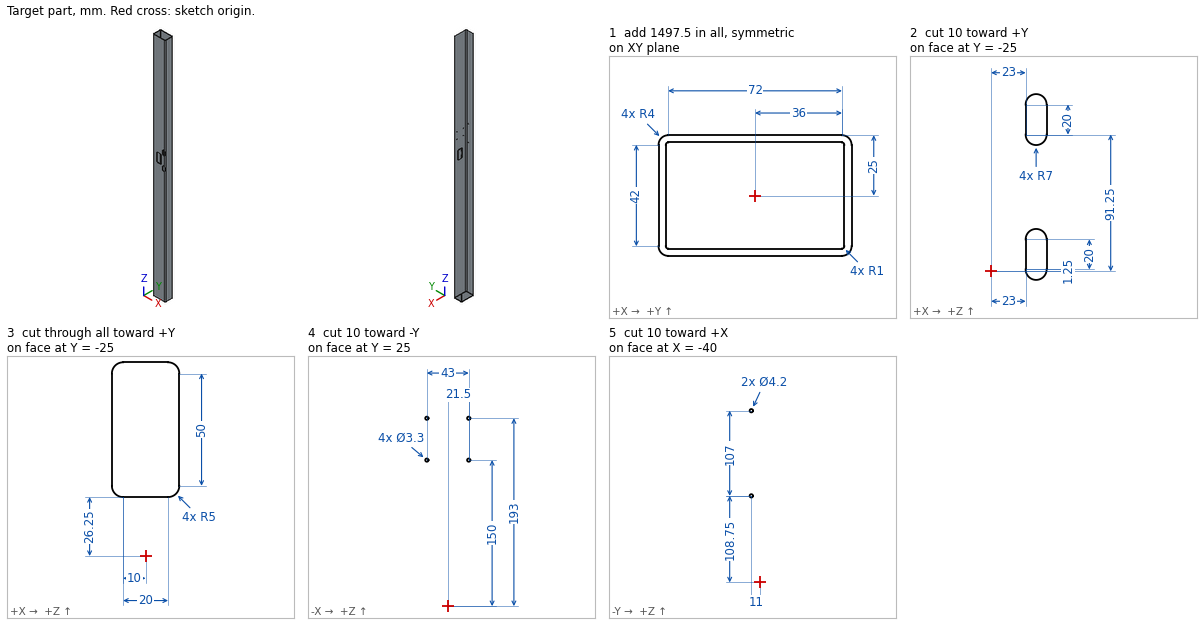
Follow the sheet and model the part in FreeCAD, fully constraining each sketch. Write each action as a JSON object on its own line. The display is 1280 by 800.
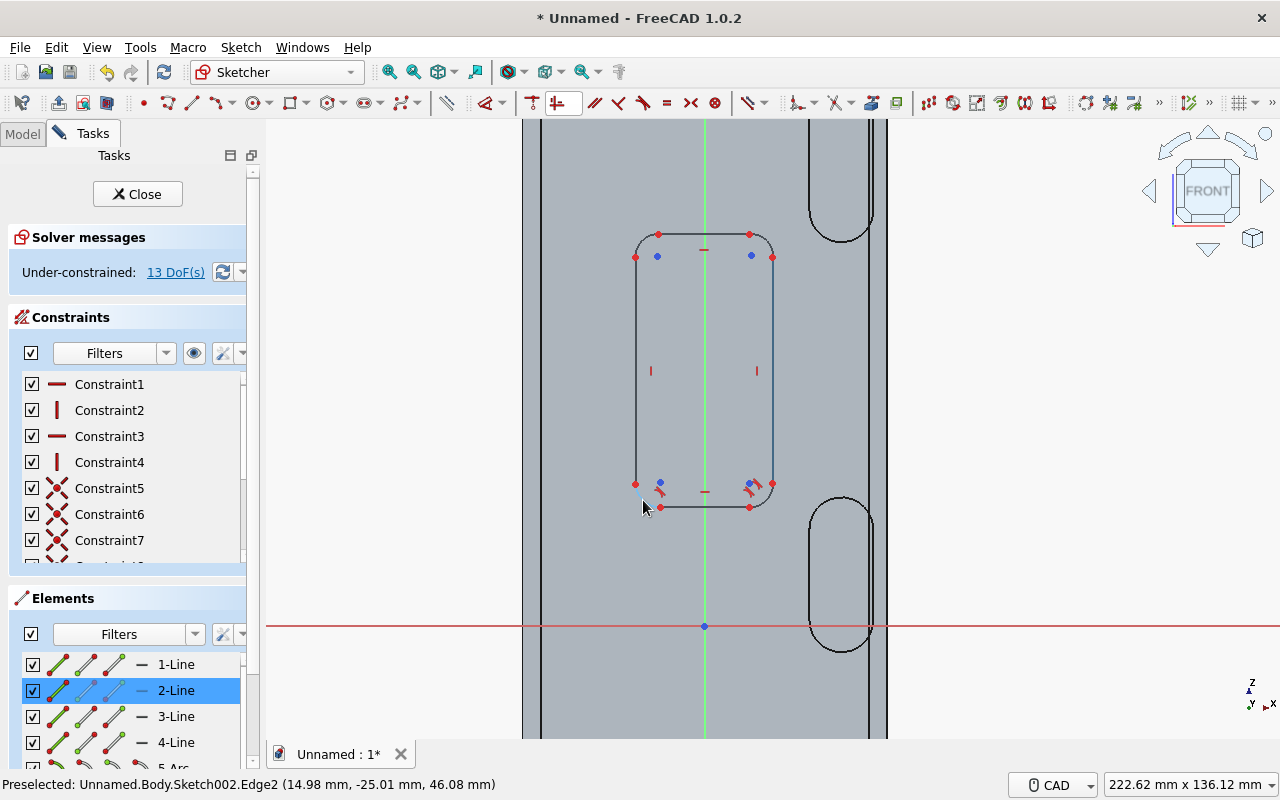
{"action": "scroll", "coordinate": [771, 247], "scroll_direction": "up", "scroll_amount": 2}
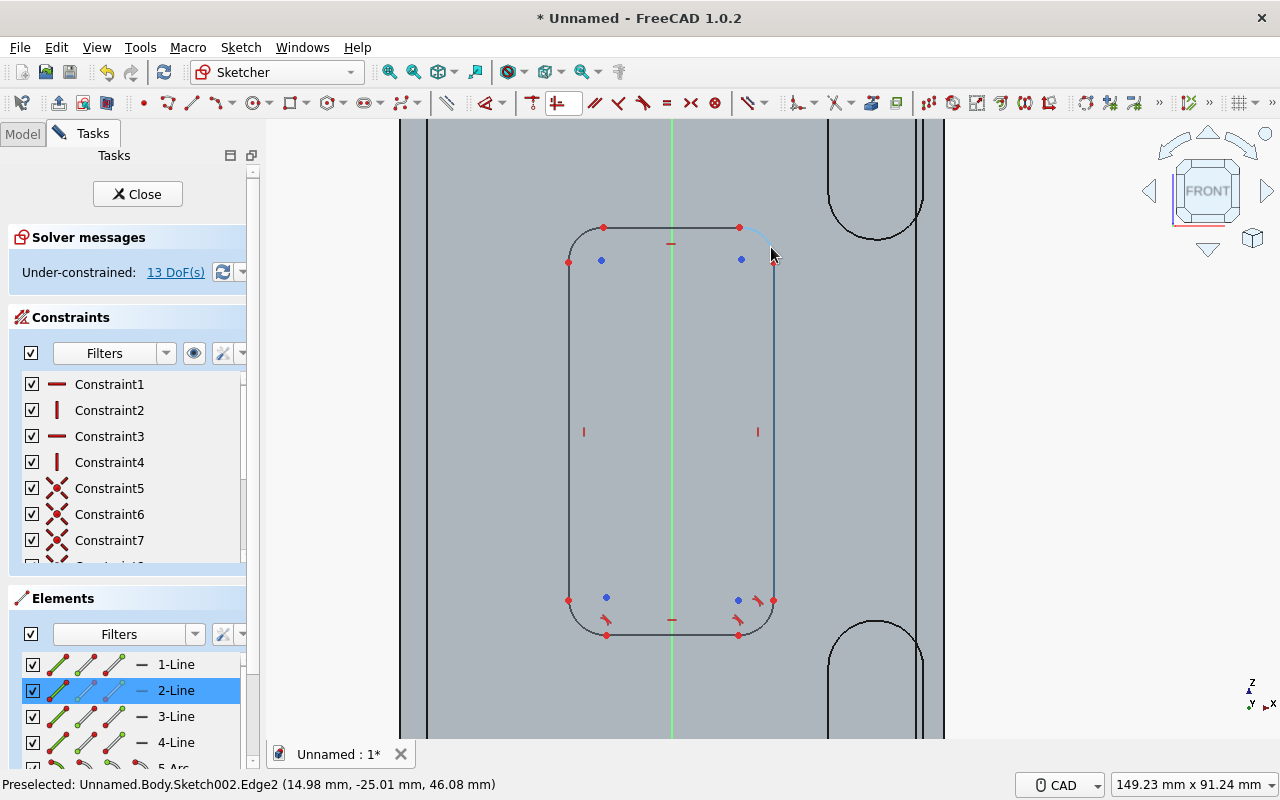
{"action": "left_click", "coordinate": [771, 246]}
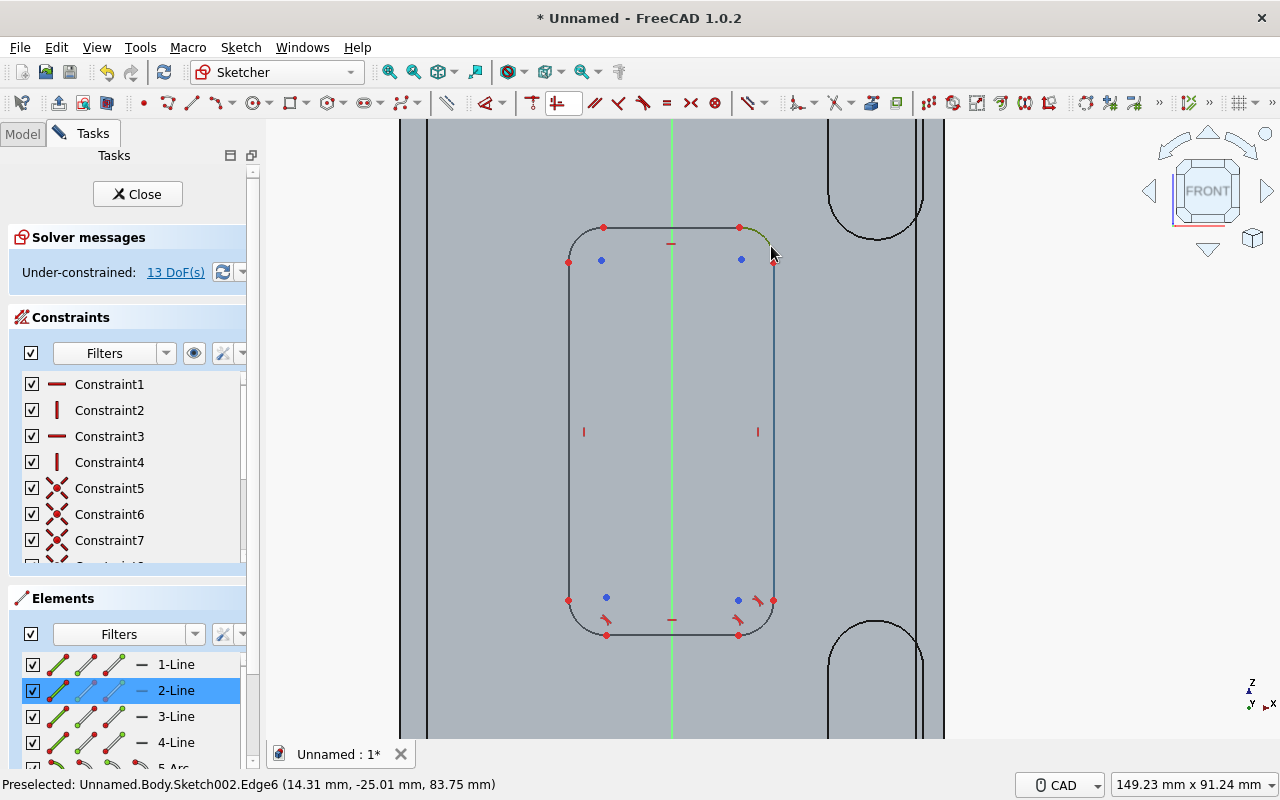
{"action": "key", "text": "t"}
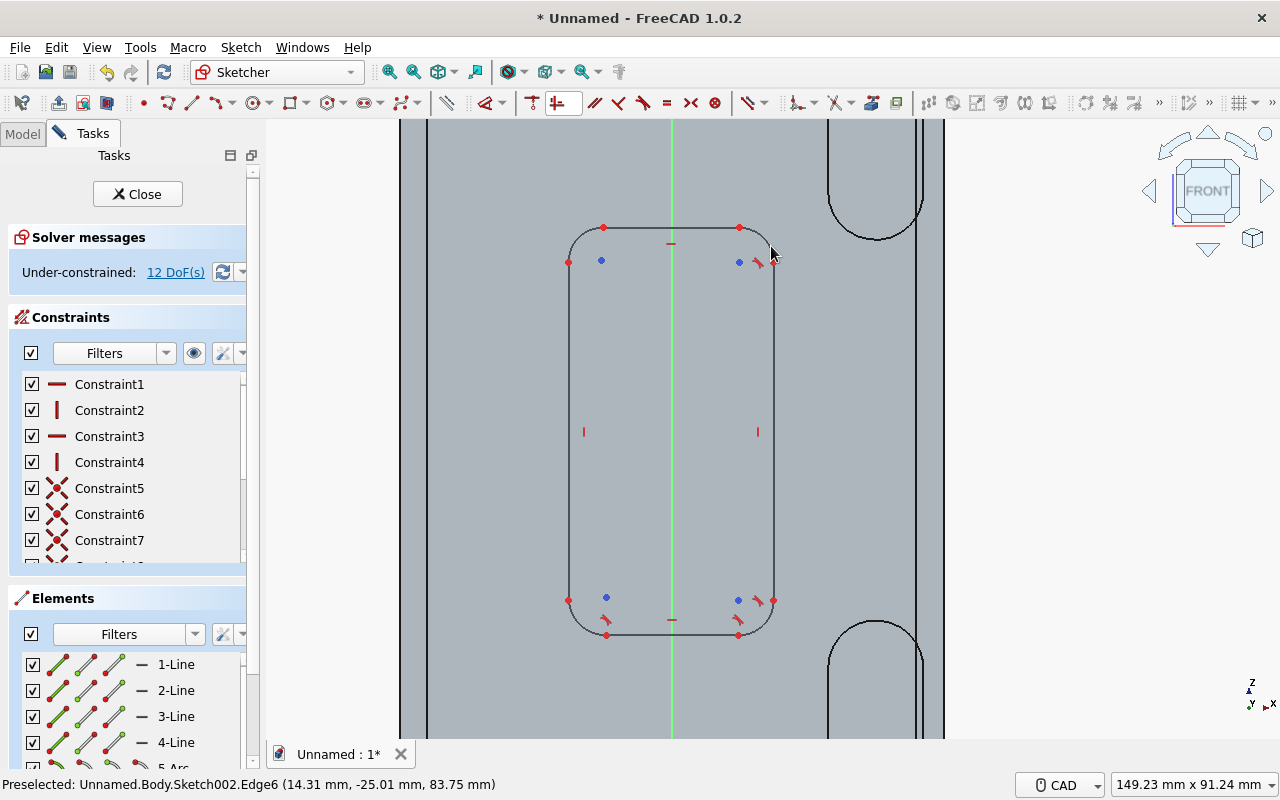
{"action": "left_click", "coordinate": [699, 228]}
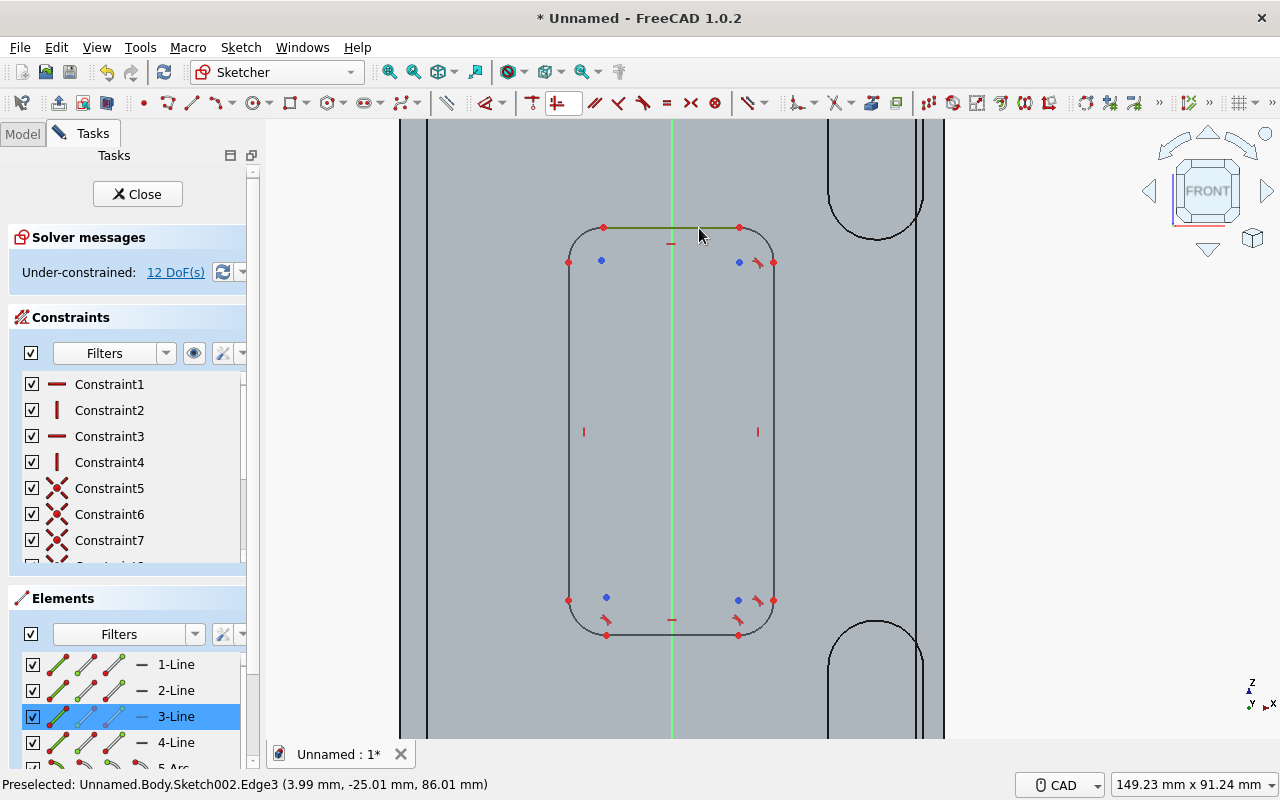
{"action": "left_click", "coordinate": [770, 247]}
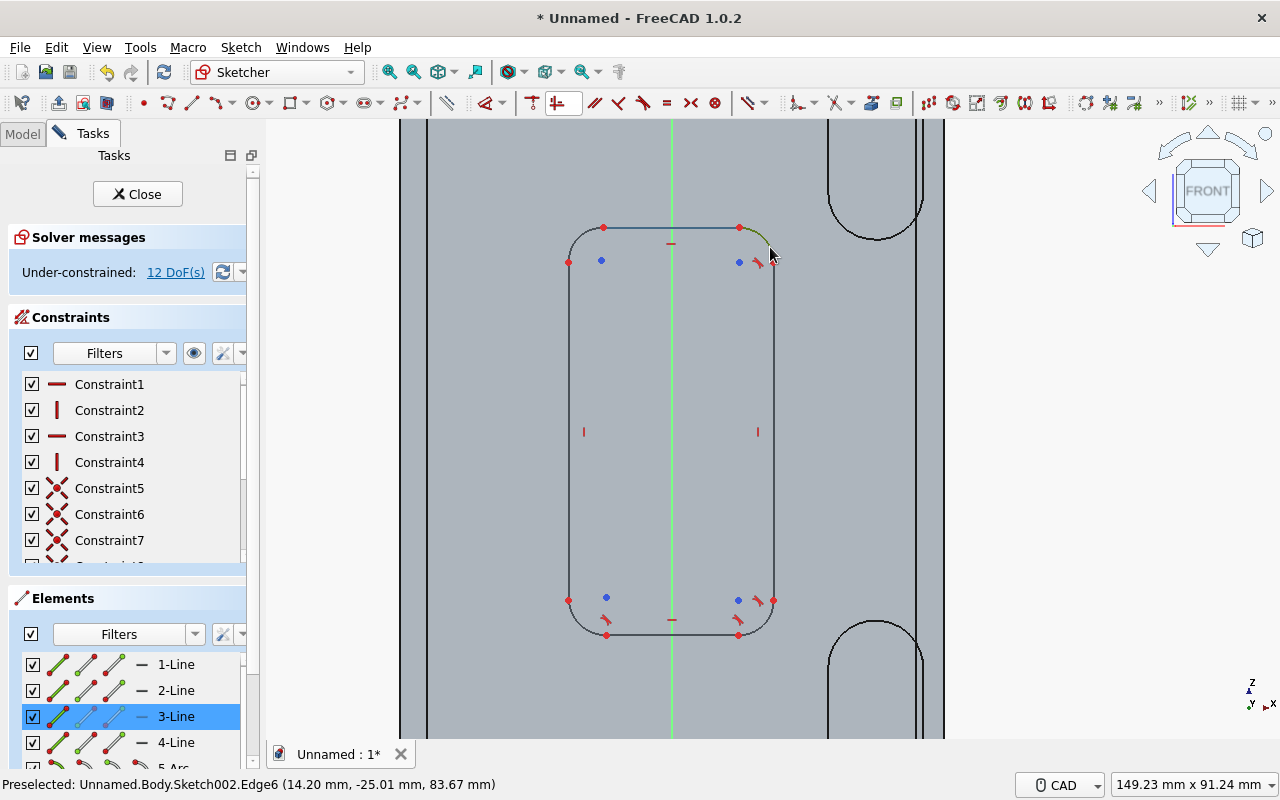
{"action": "key", "text": "t"}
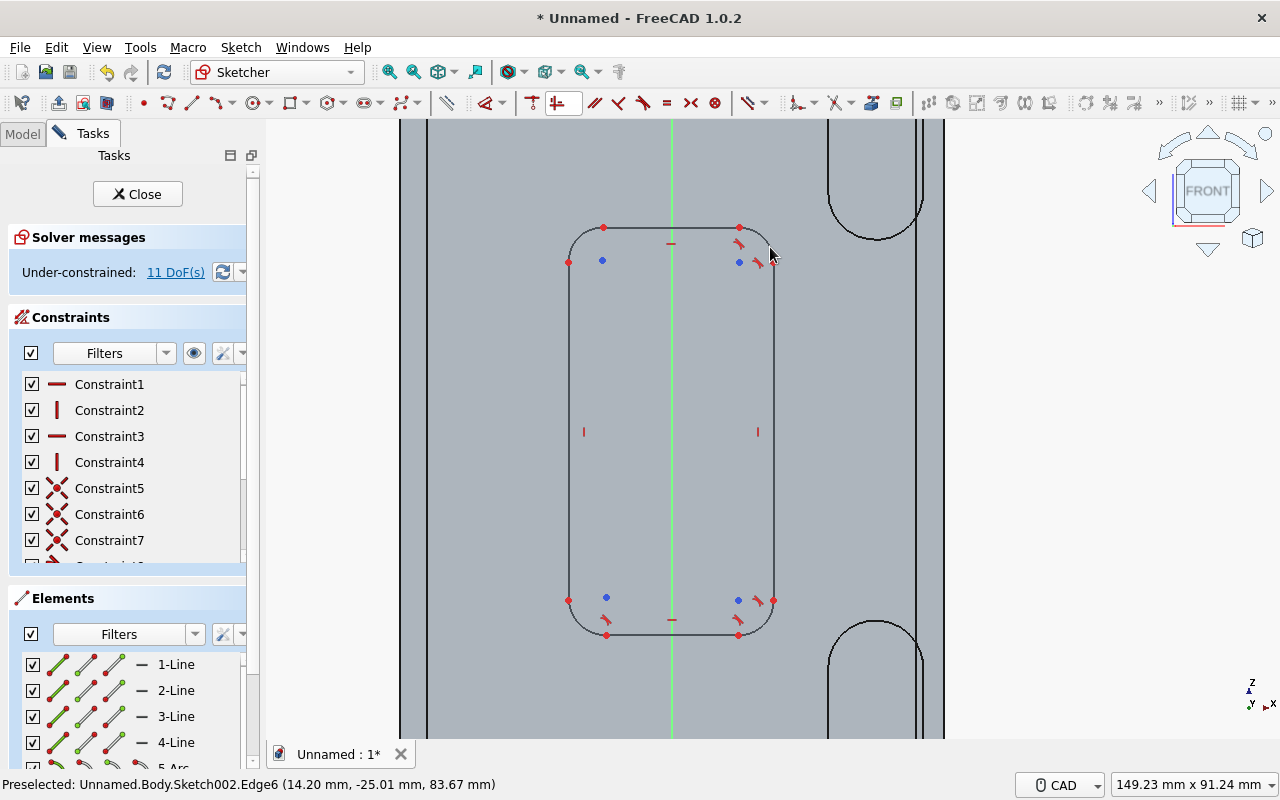
{"action": "left_click", "coordinate": [699, 228]}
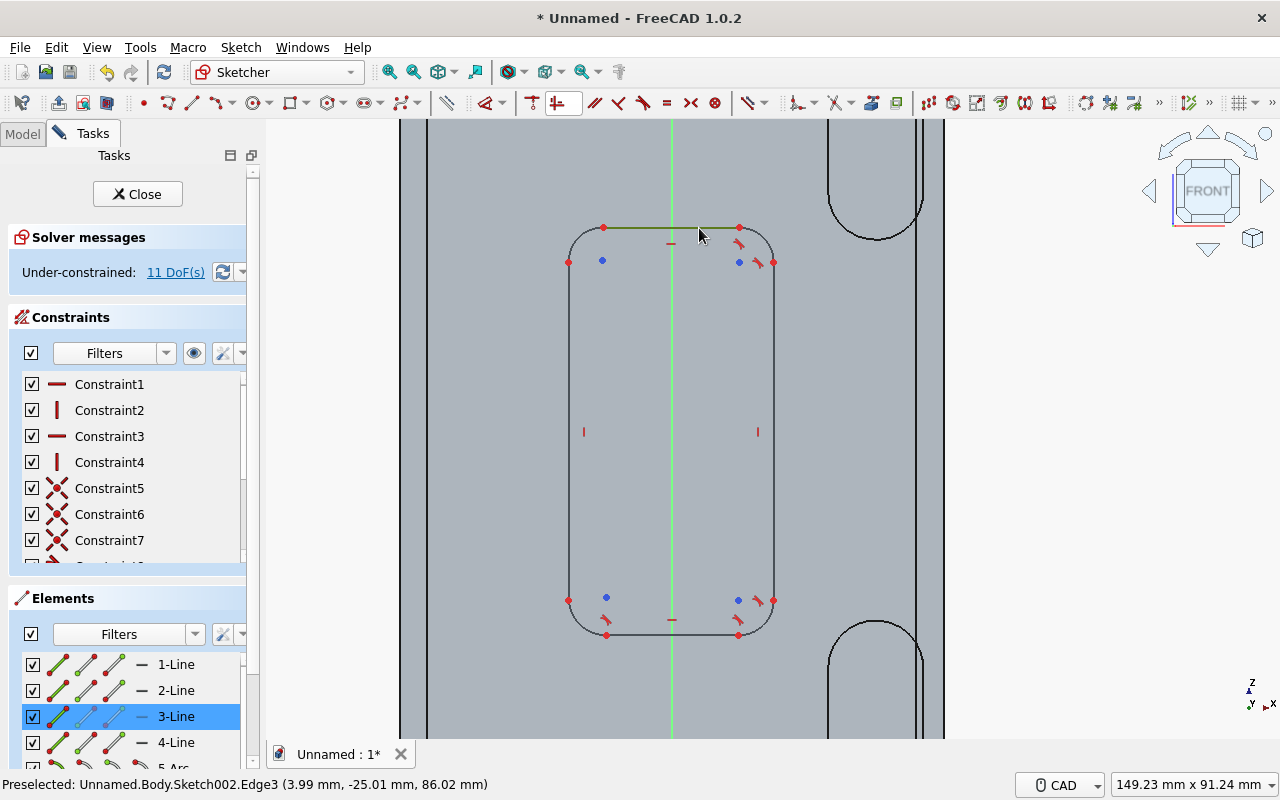
{"action": "left_click", "coordinate": [588, 231]}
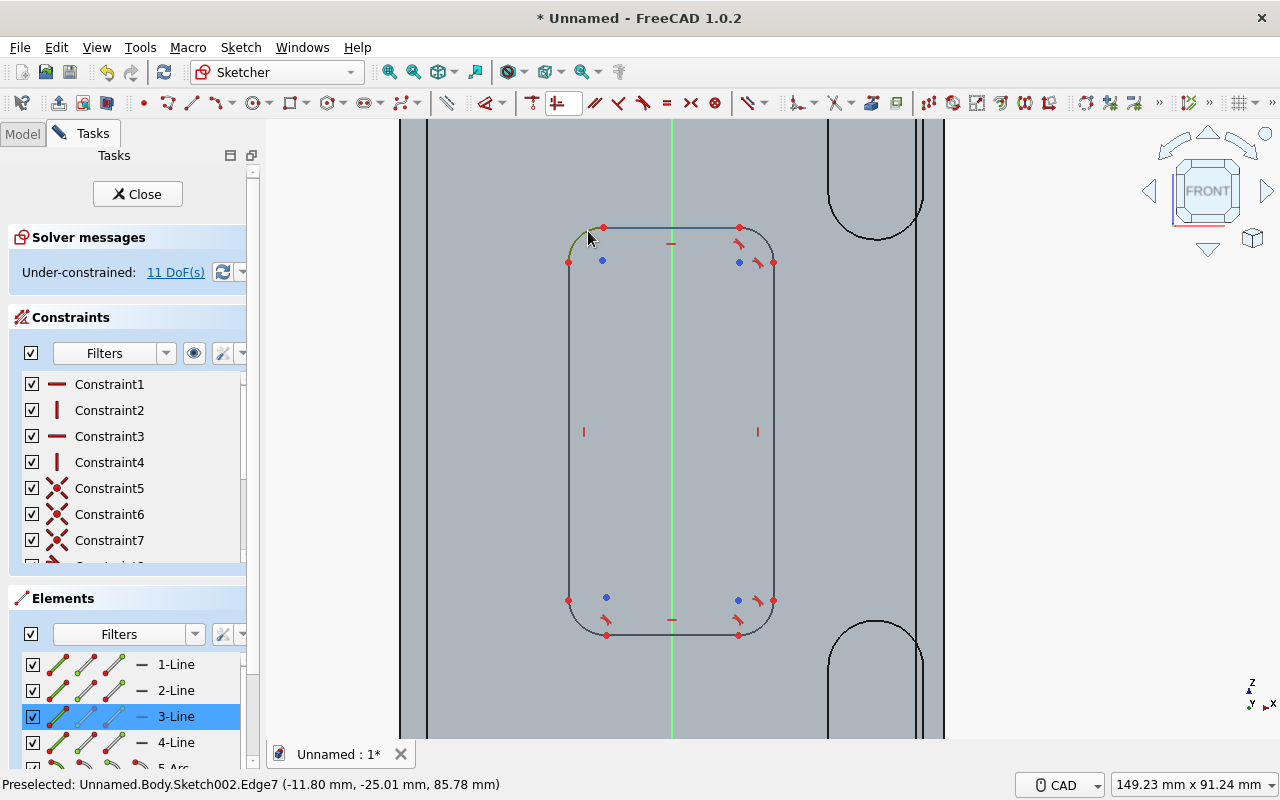
{"action": "key", "text": "t"}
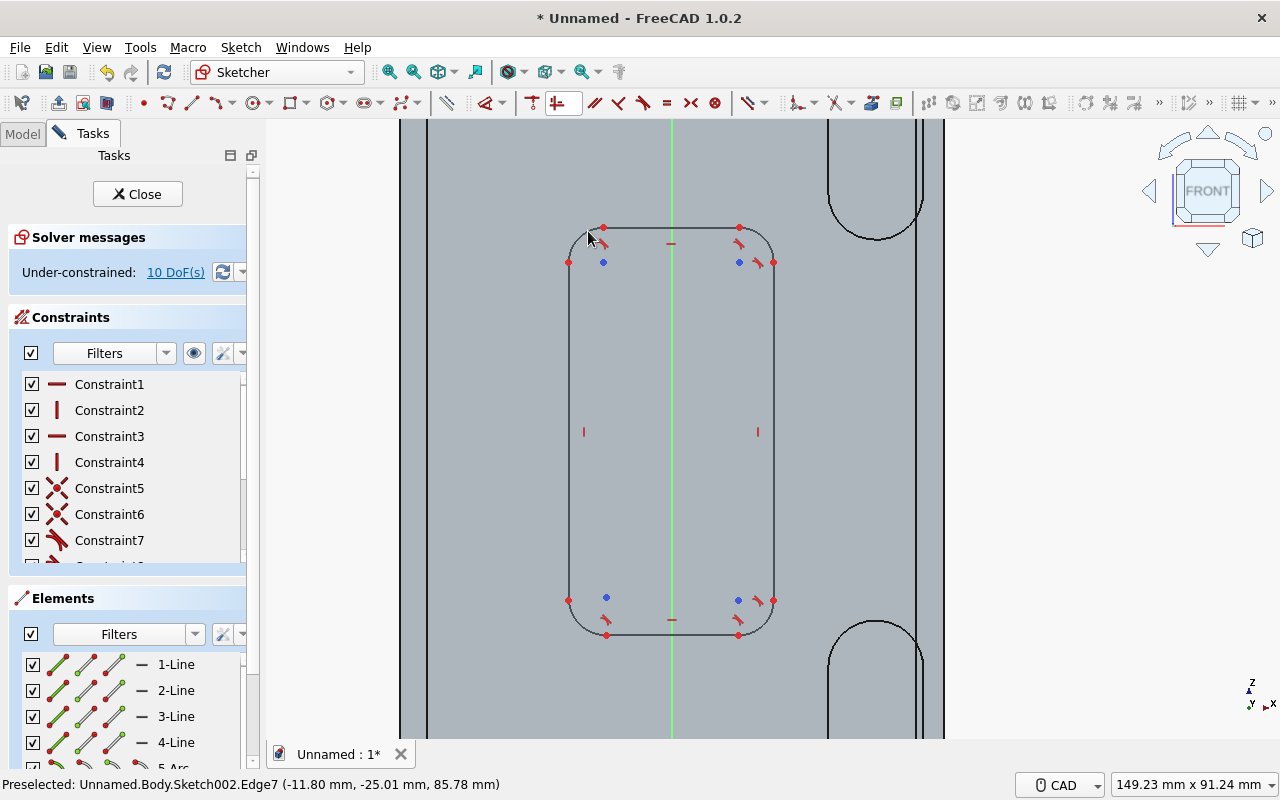
{"action": "left_click", "coordinate": [569, 364]}